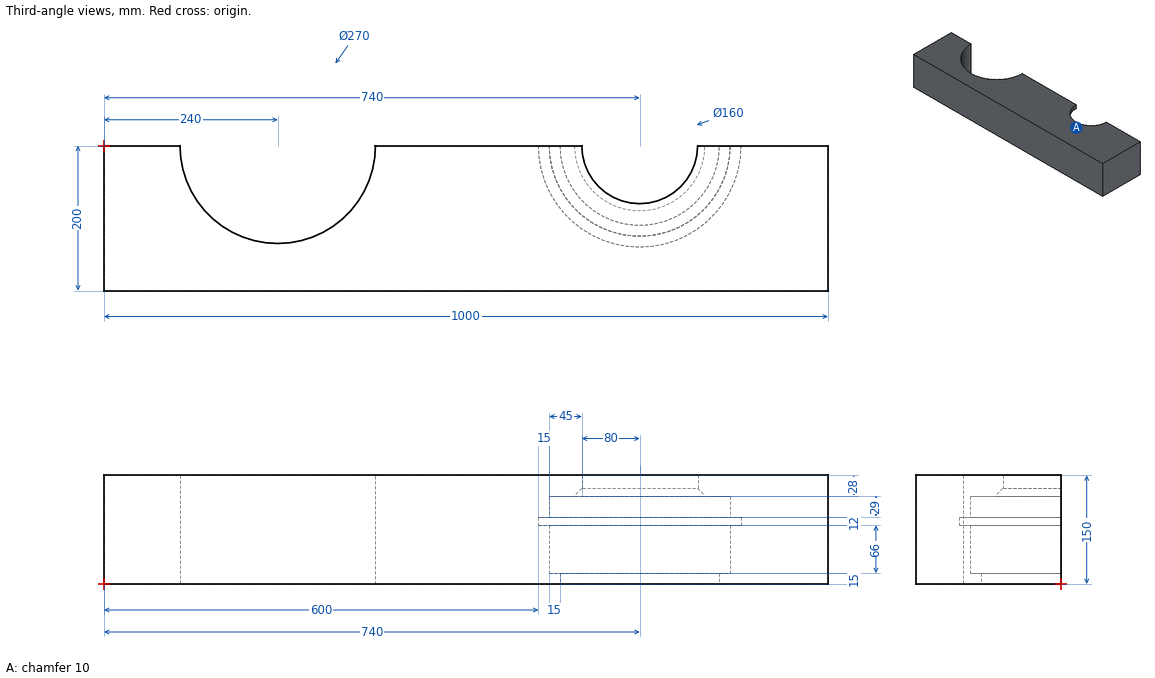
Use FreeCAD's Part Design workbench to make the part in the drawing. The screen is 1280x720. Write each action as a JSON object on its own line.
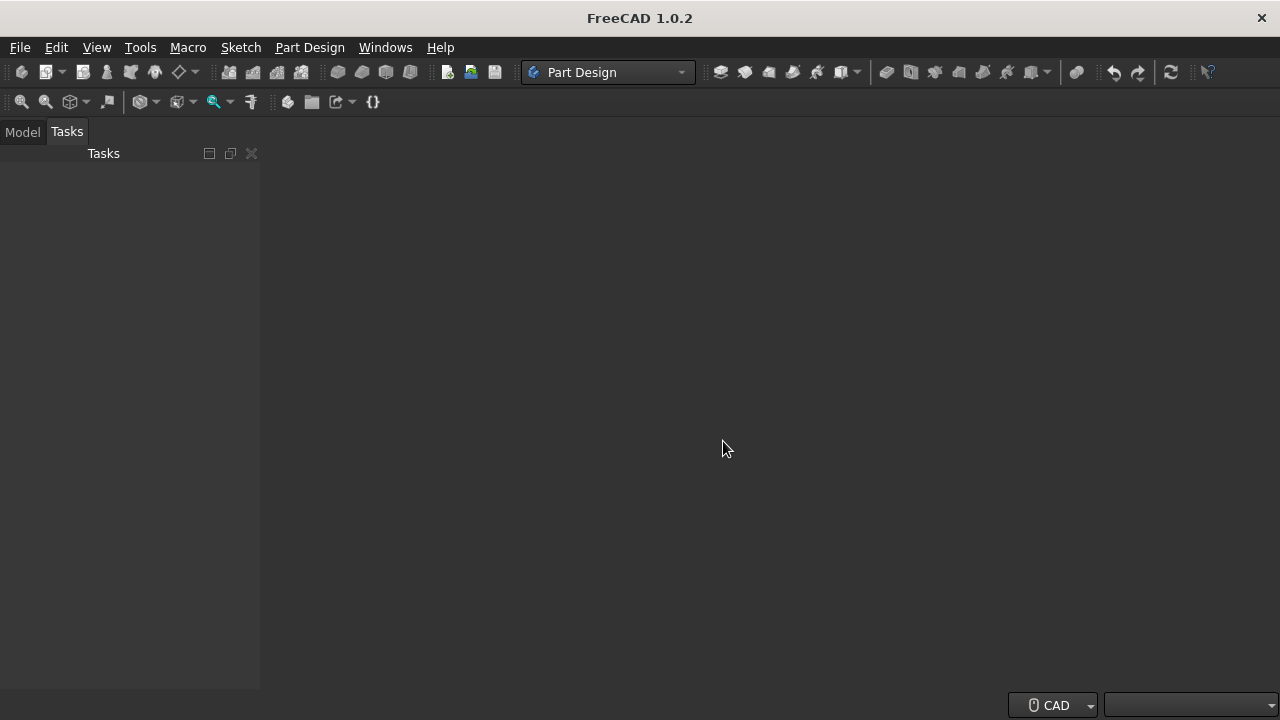
{"action": "left_click", "coordinate": [448, 72]}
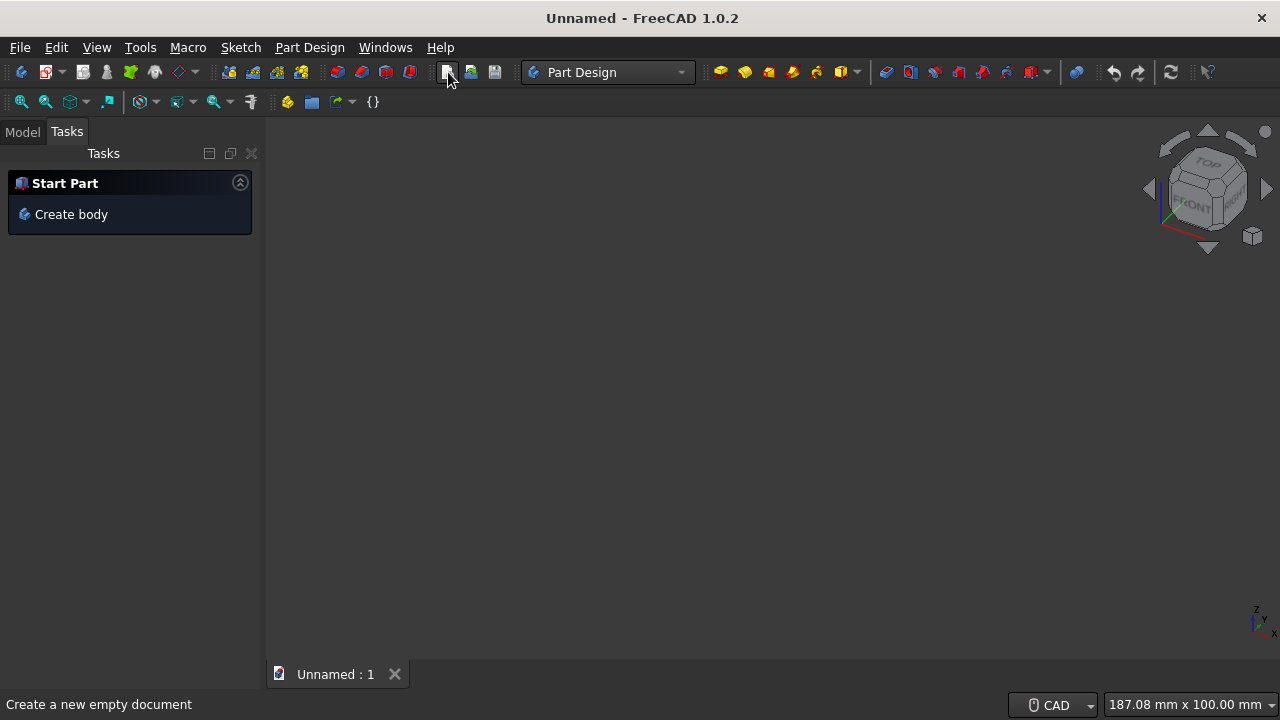
{"action": "left_click", "coordinate": [46, 72]}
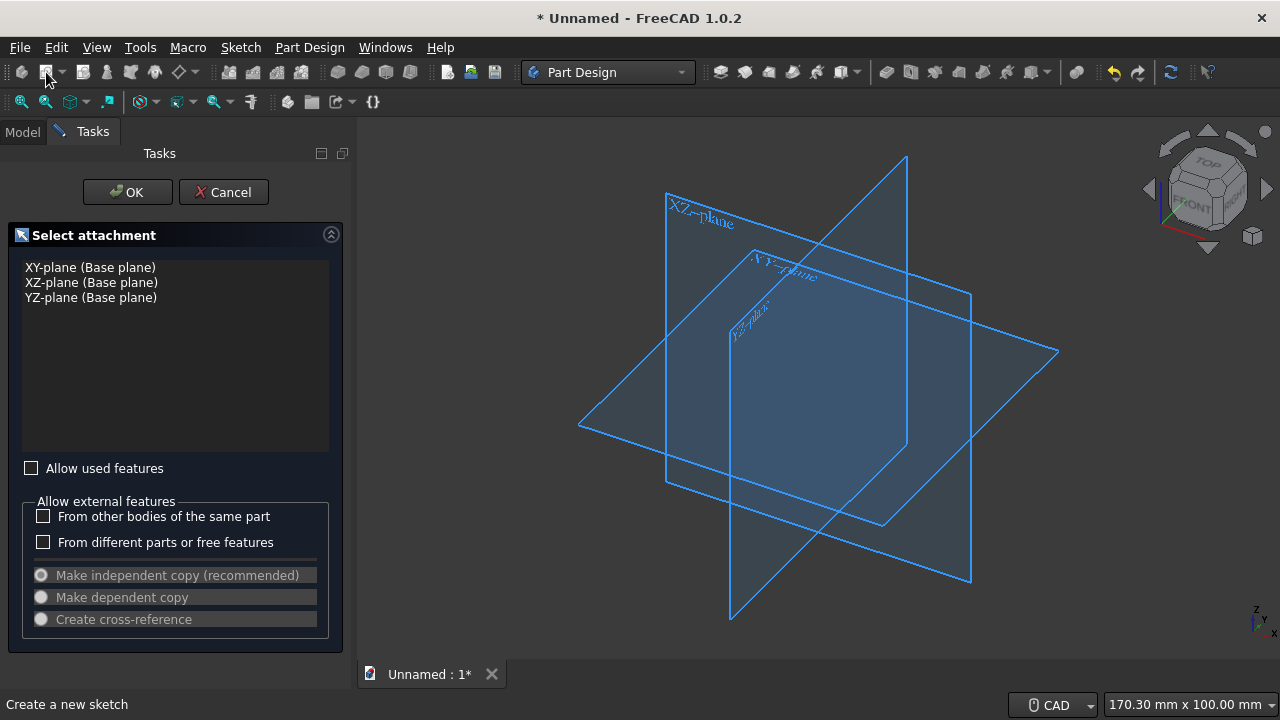
{"action": "left_click", "coordinate": [82, 268]}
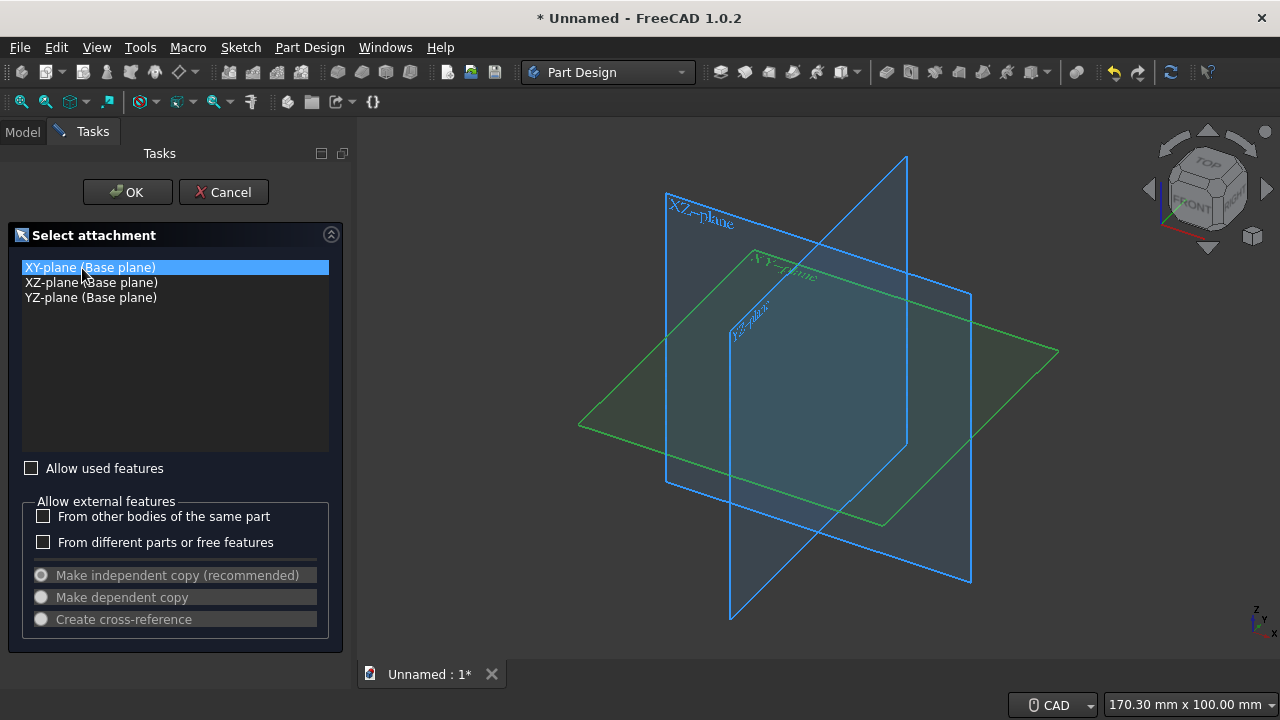
{"action": "left_click", "coordinate": [128, 192]}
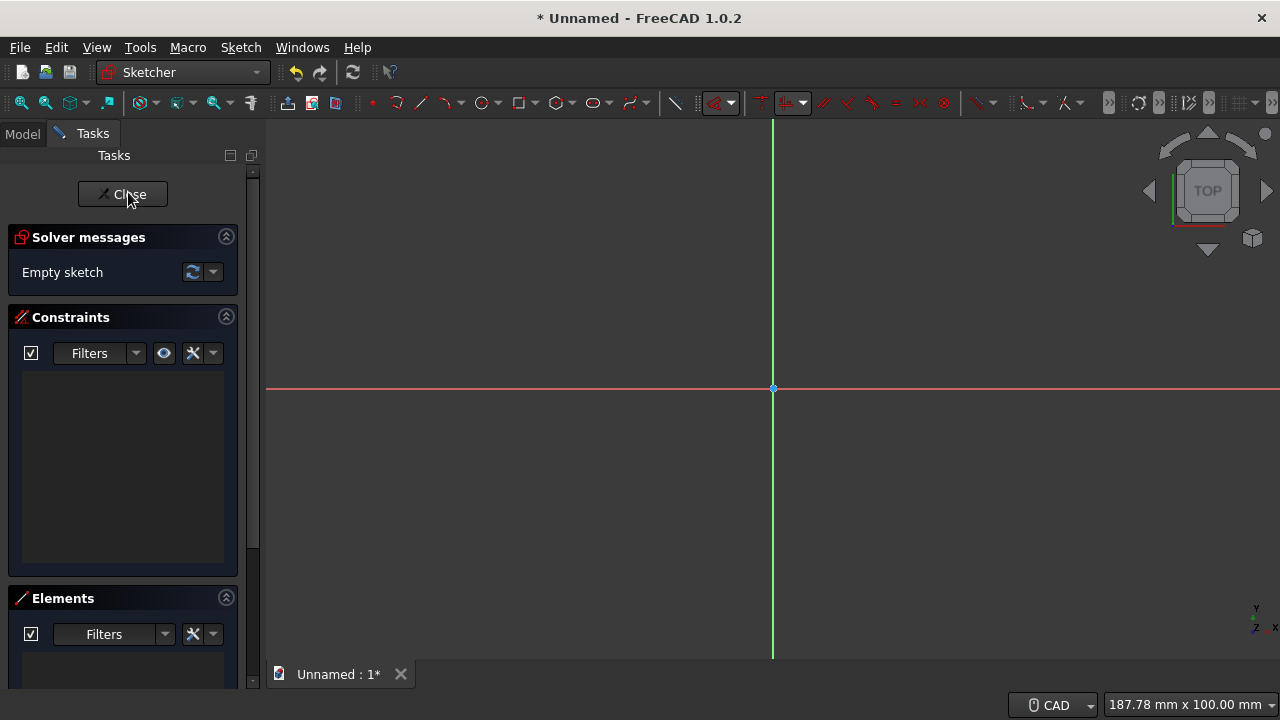
{"action": "scroll", "coordinate": [360, 322], "scroll_direction": "down", "scroll_amount": 11}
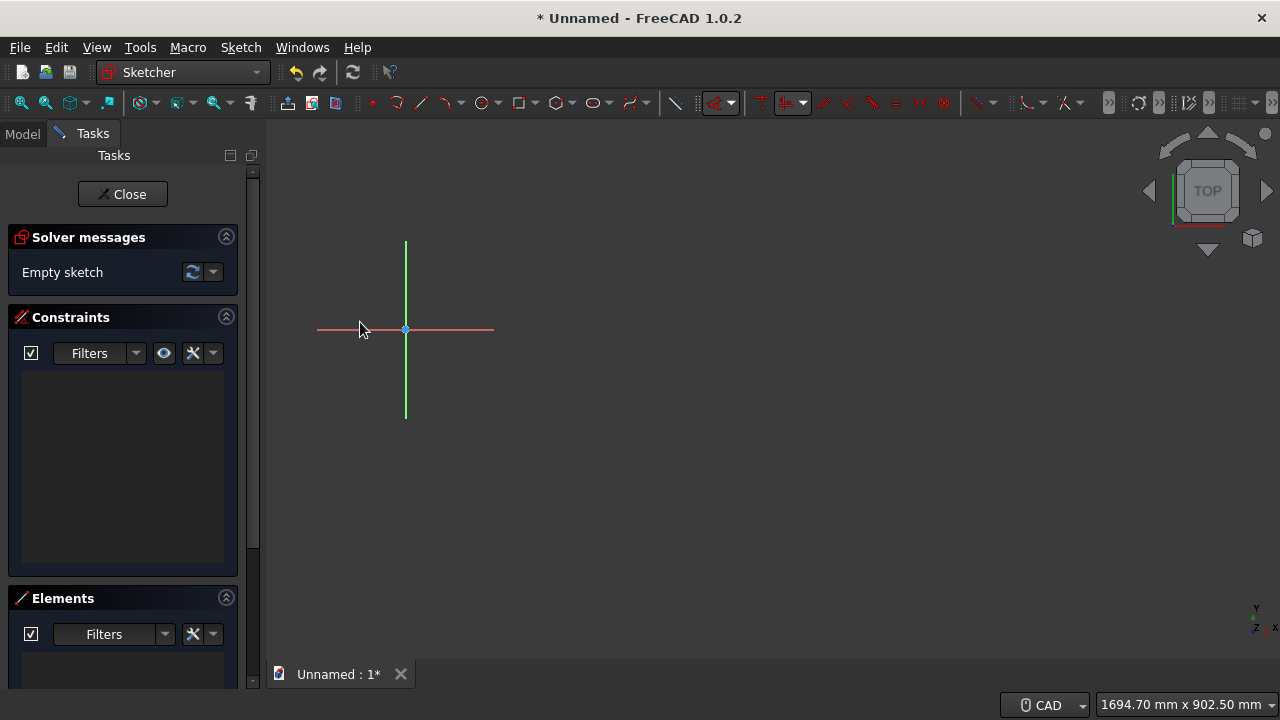
{"action": "left_click", "coordinate": [520, 104]}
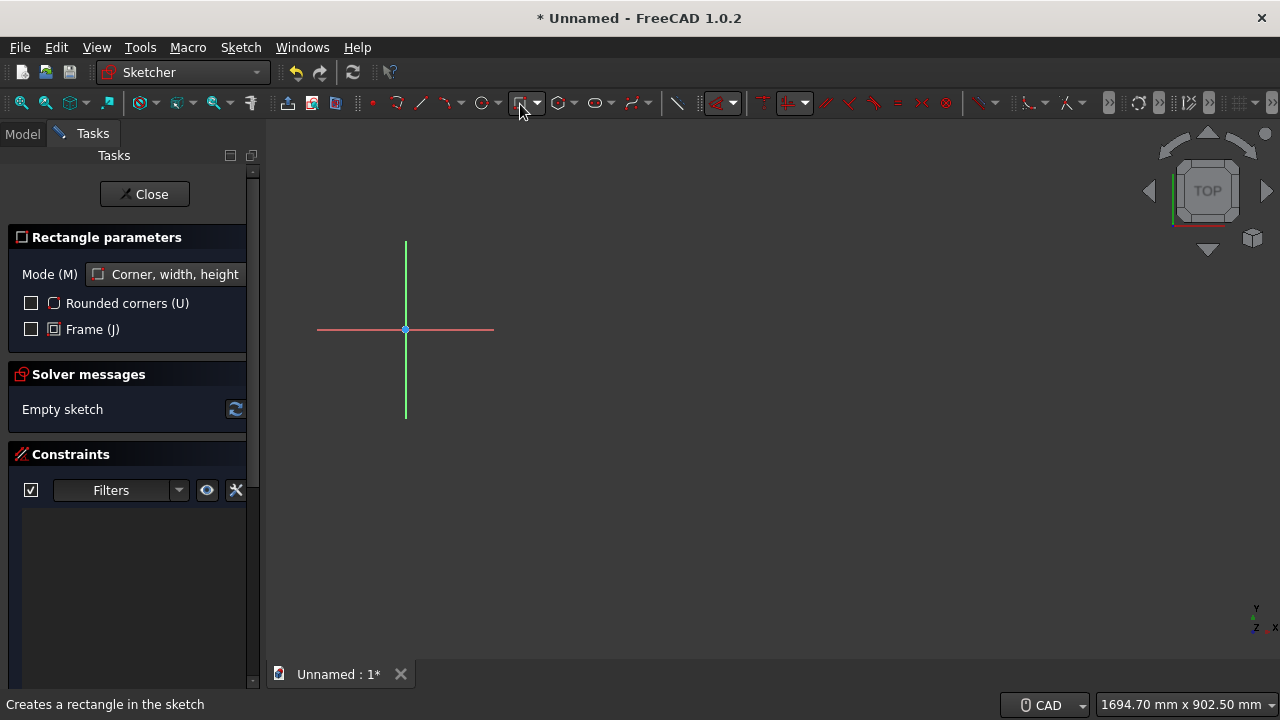
{"action": "left_click", "coordinate": [406, 330]}
{"action": "left_click", "coordinate": [1004, 449]}
{"action": "key", "text": "Escape"}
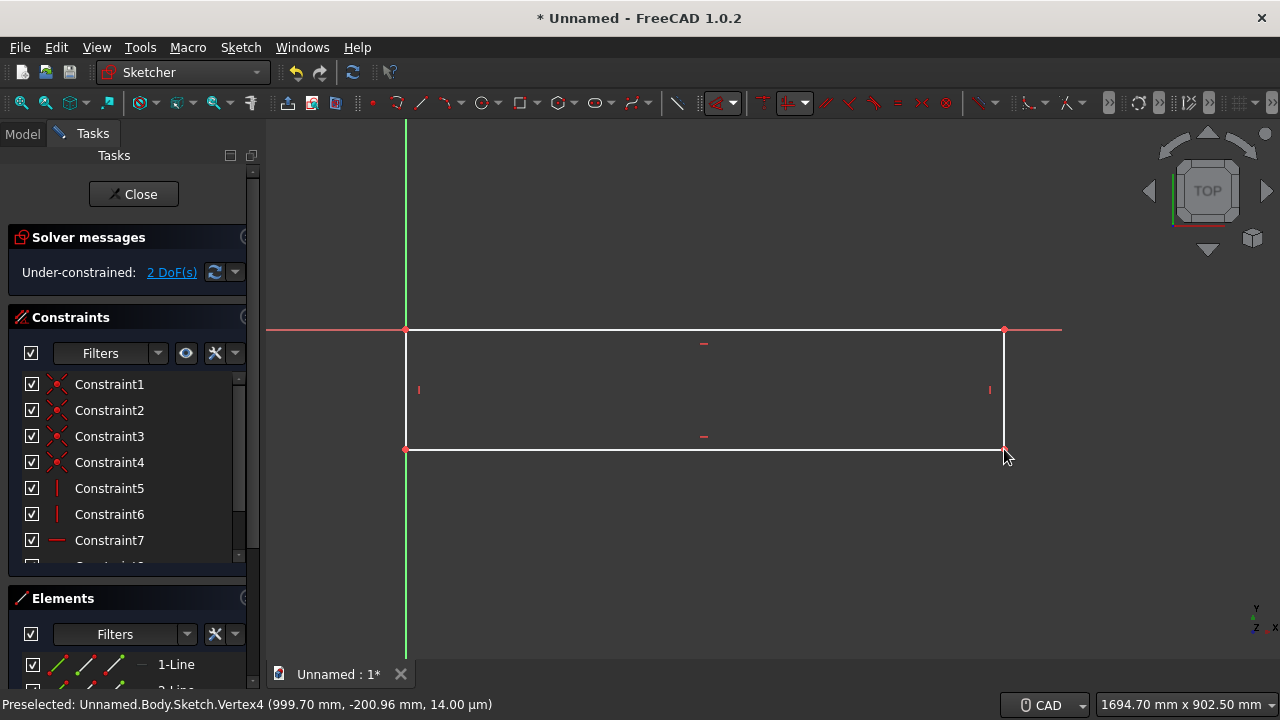
{"action": "left_click", "coordinate": [716, 104]}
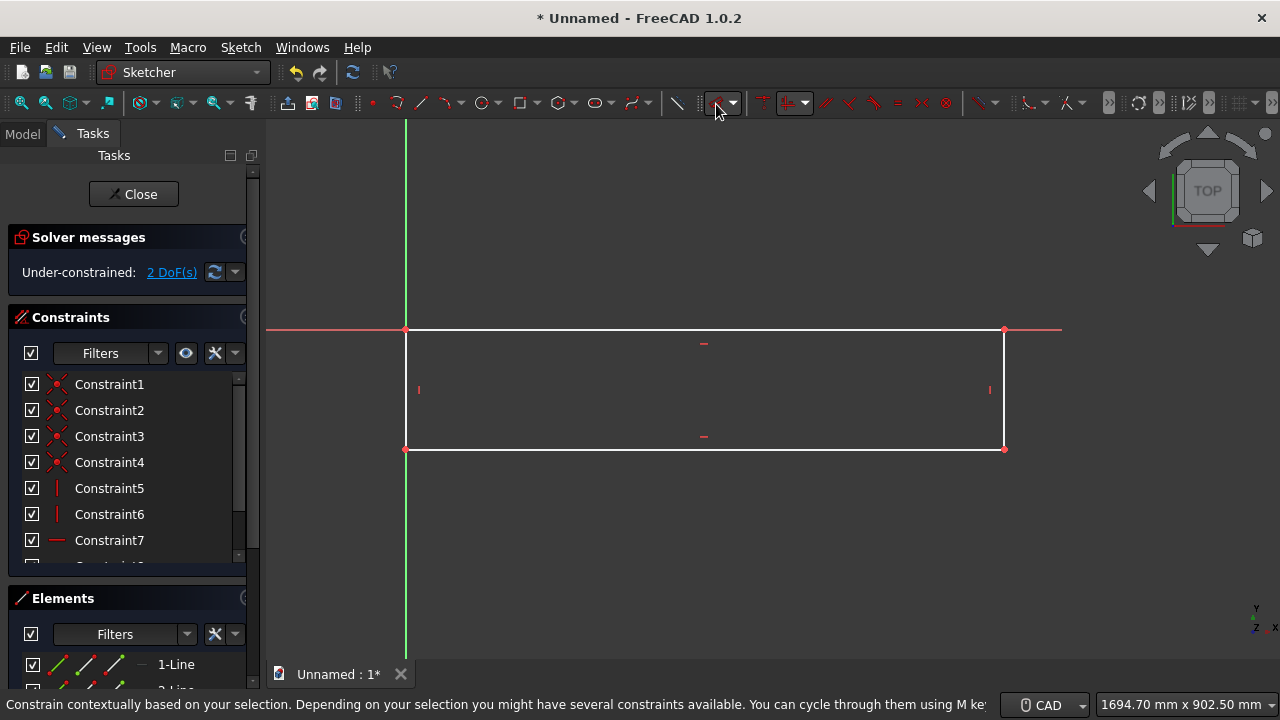
{"action": "left_click", "coordinate": [406, 366]}
{"action": "left_click", "coordinate": [372, 390]}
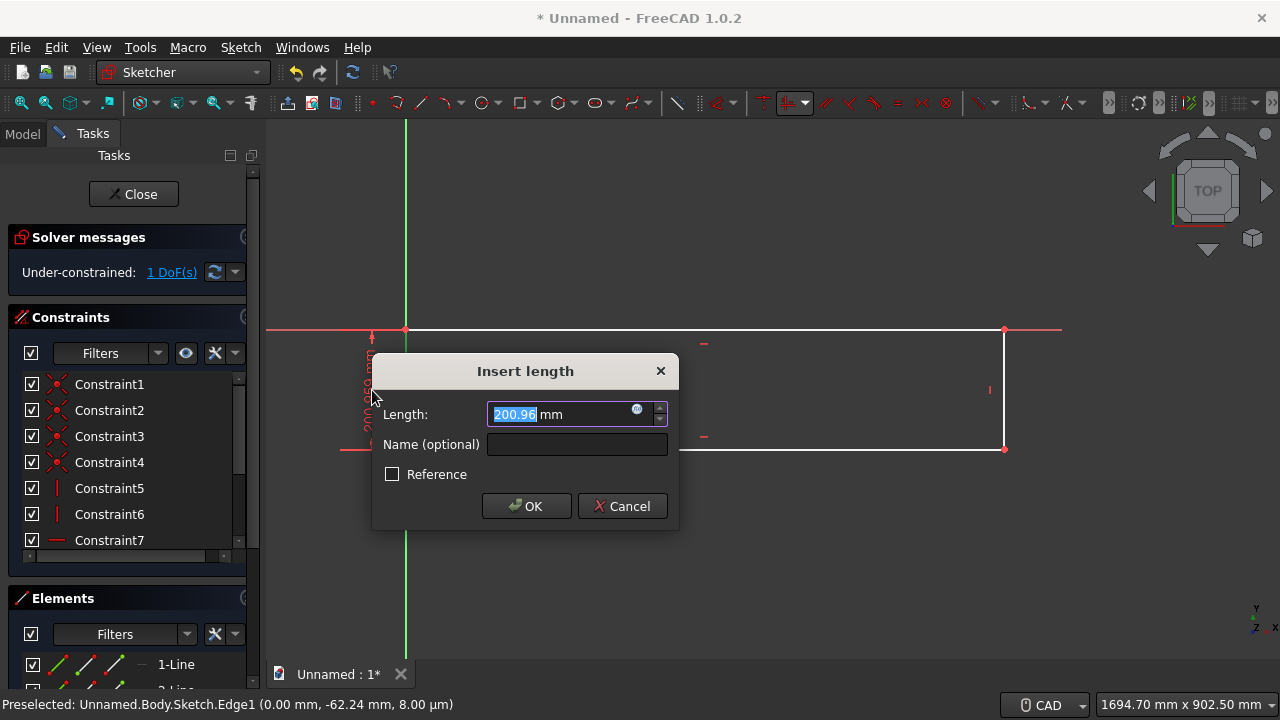
{"action": "type", "text": "200"}
{"action": "key", "text": "Return"}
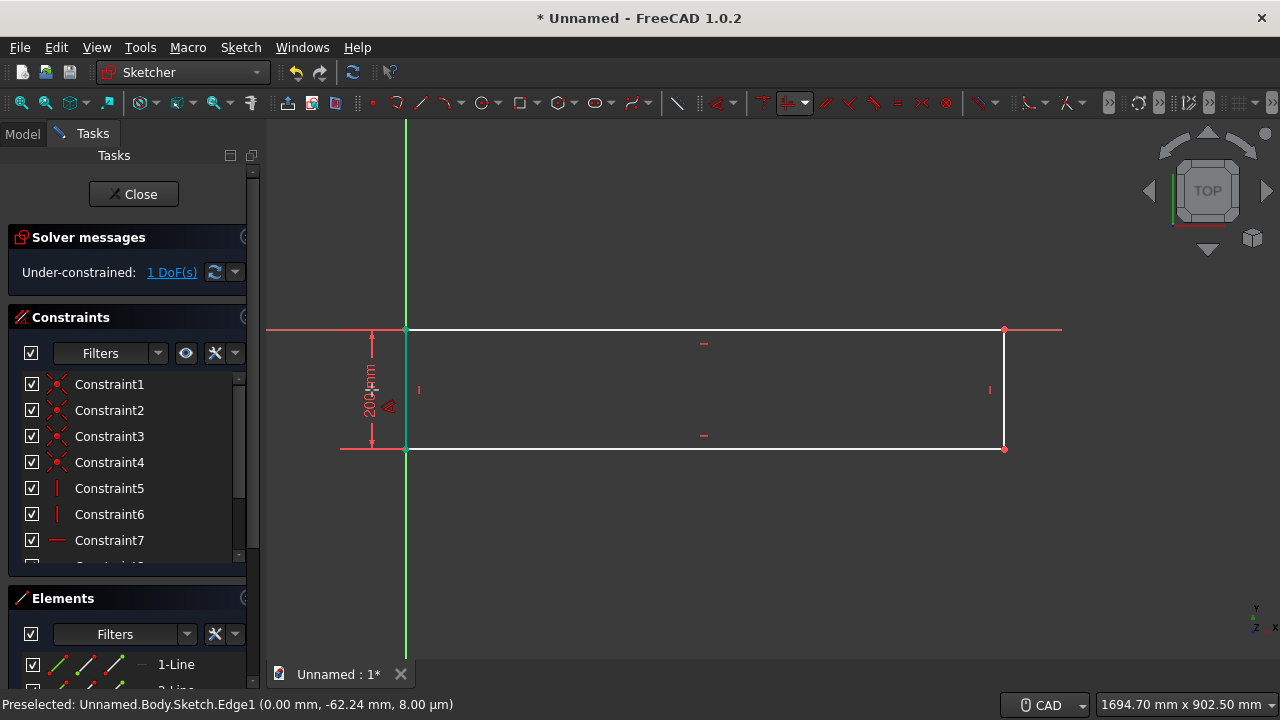
{"action": "left_click", "coordinate": [585, 449]}
{"action": "left_click", "coordinate": [705, 483]}